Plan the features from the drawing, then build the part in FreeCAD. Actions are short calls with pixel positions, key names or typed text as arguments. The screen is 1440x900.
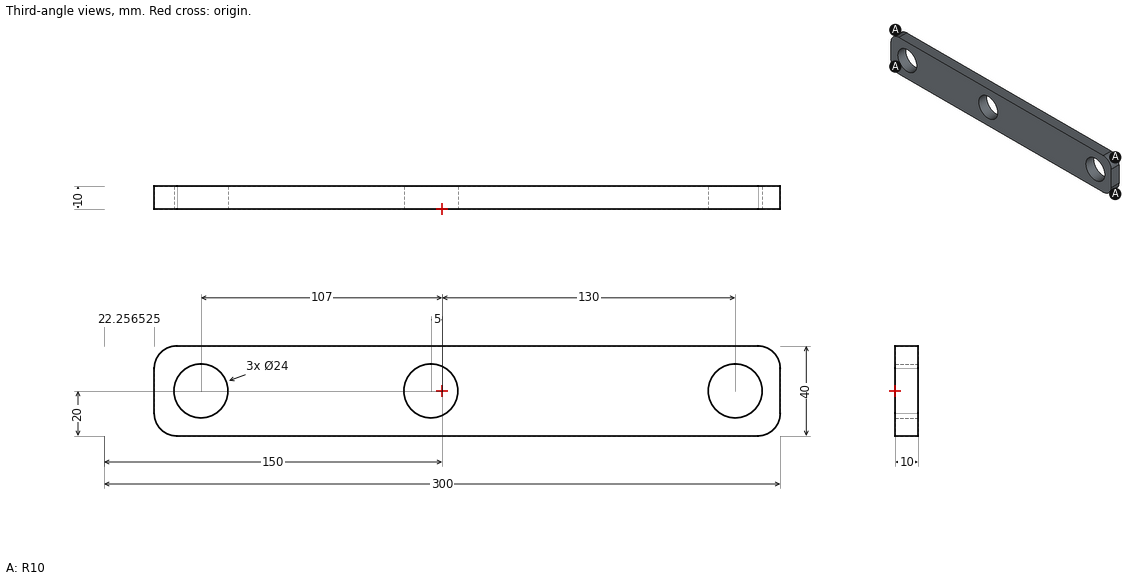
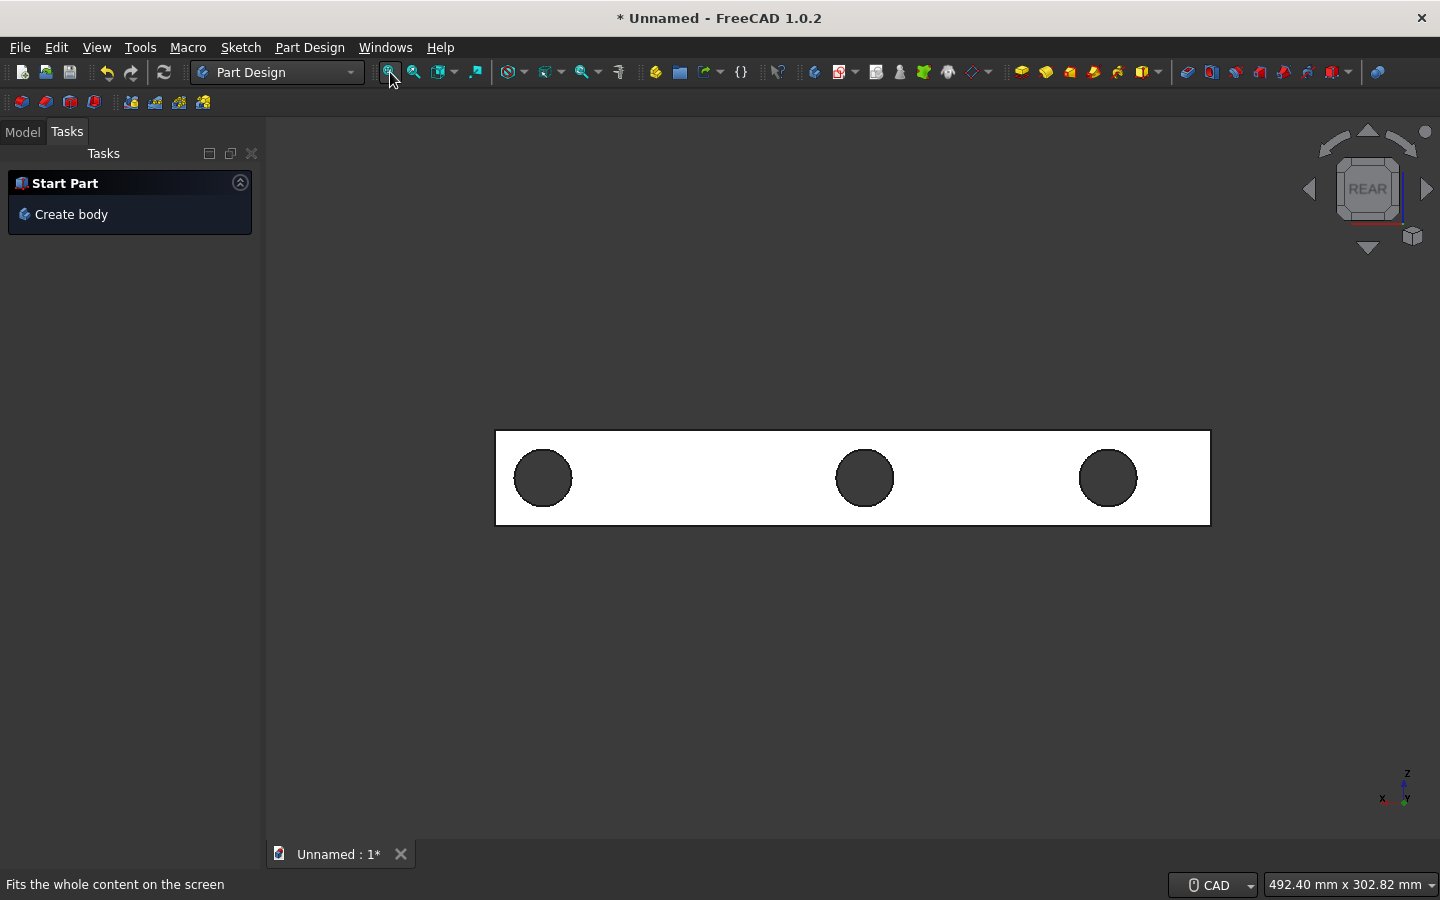
click(649, 477)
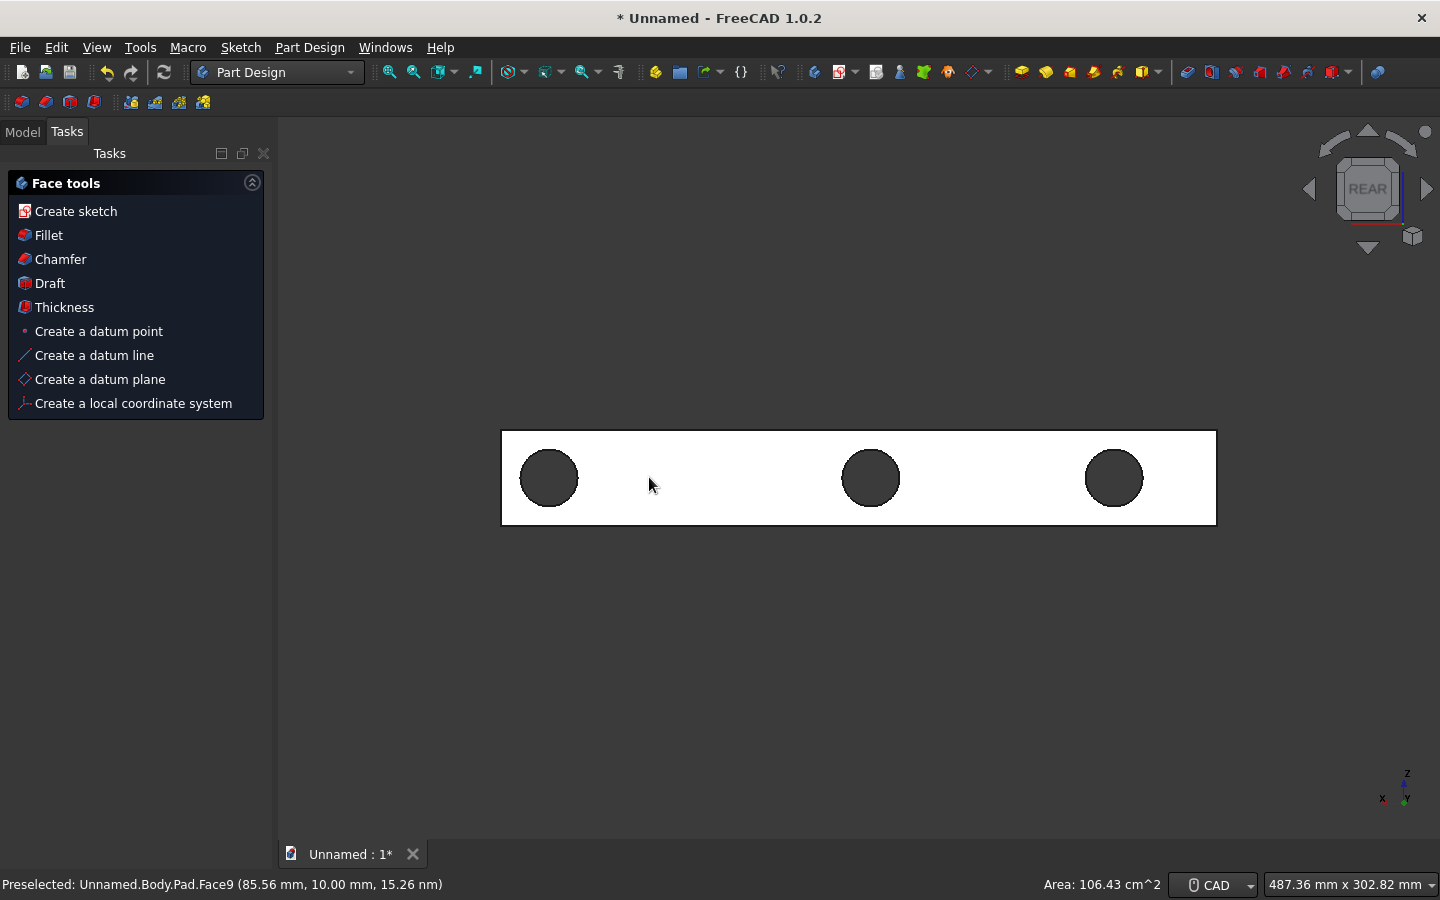
click(840, 72)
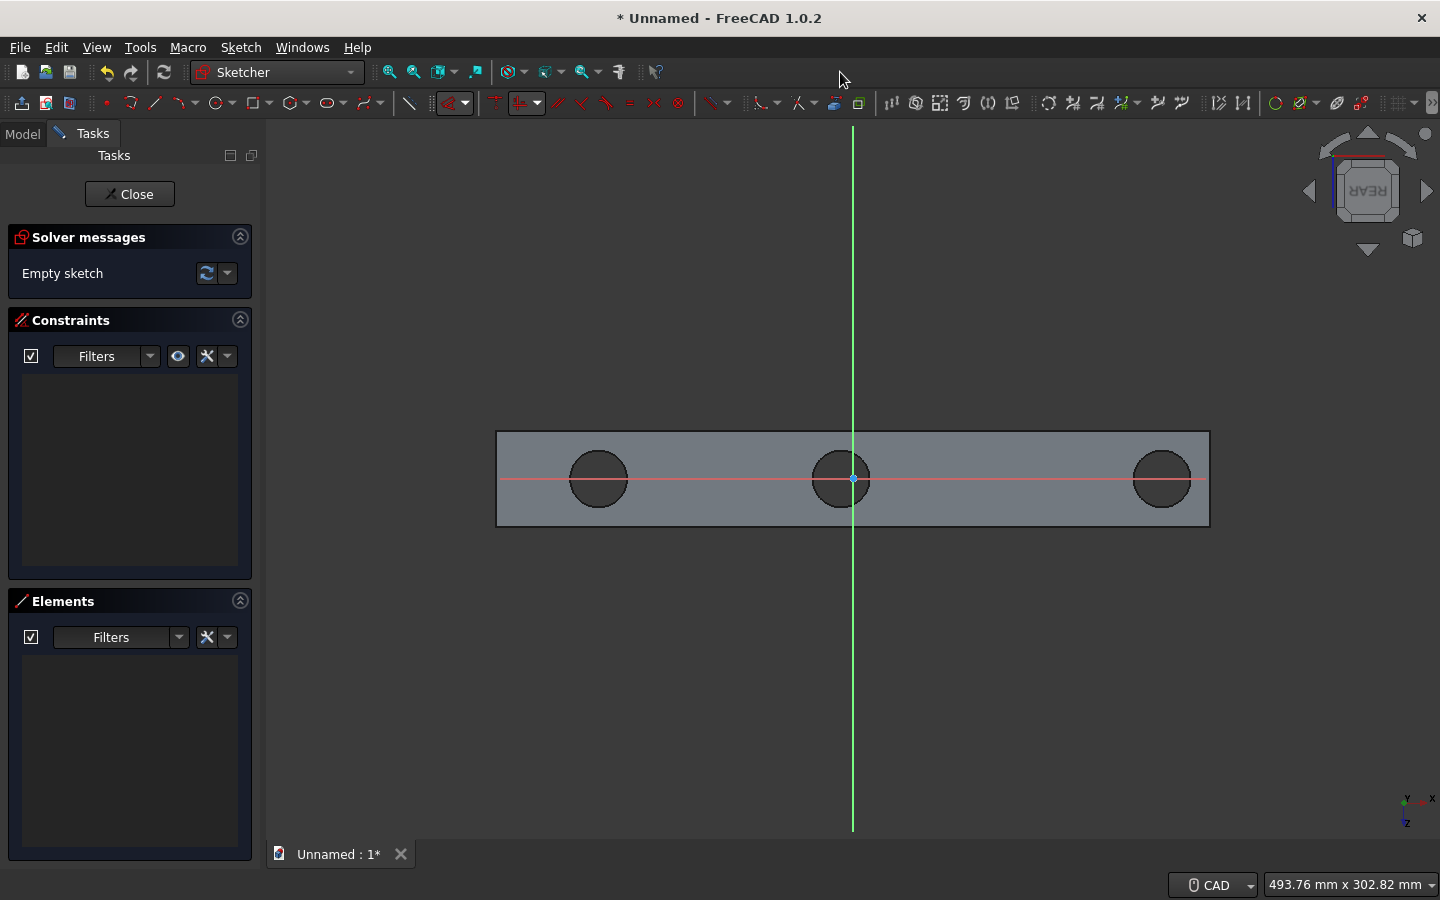
scroll(457, 479, up, 8)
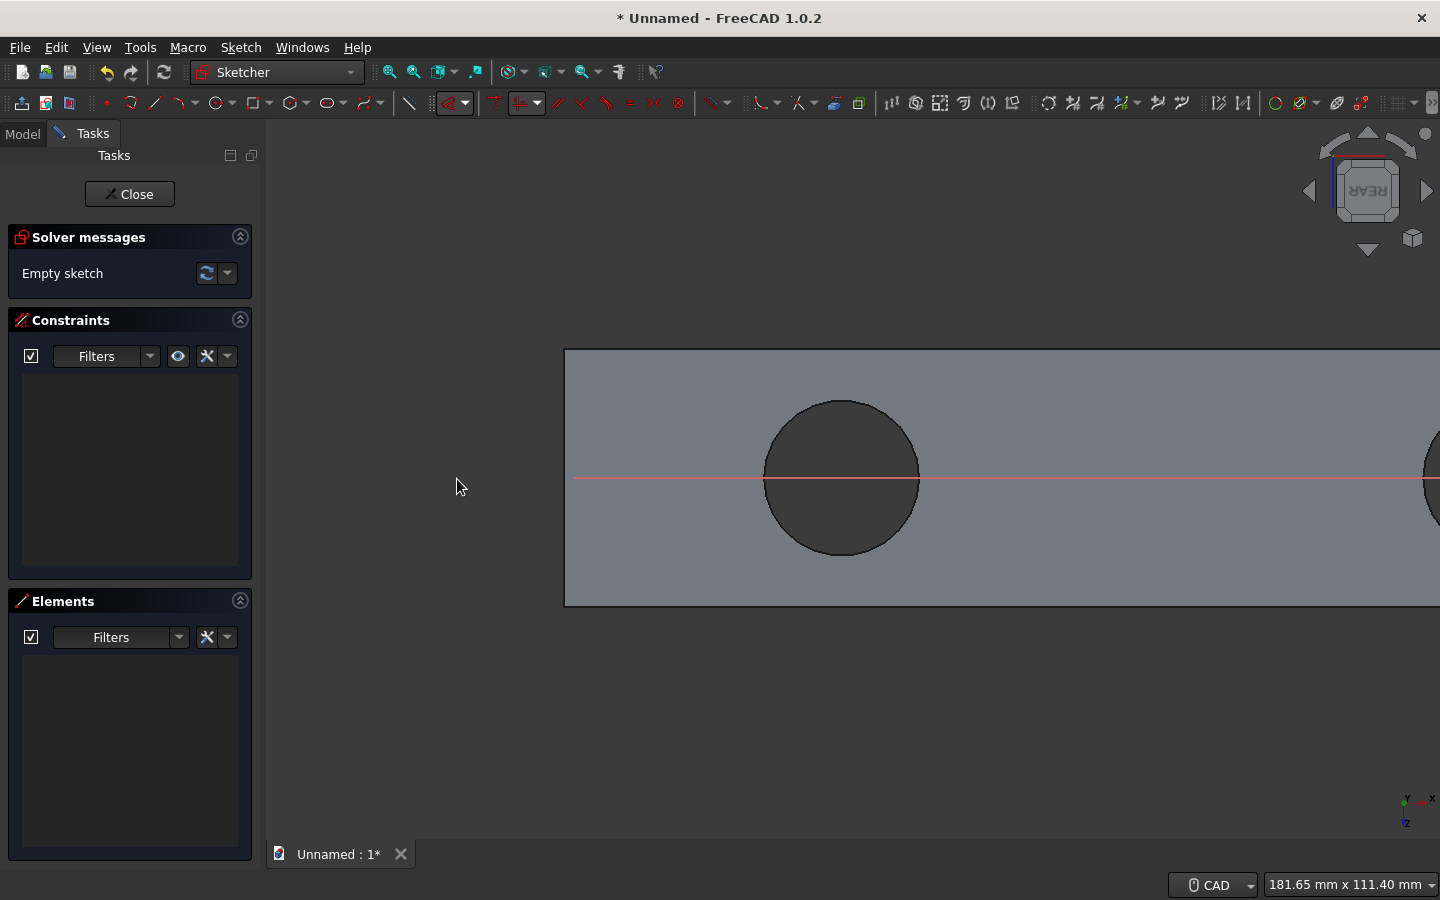
click(254, 104)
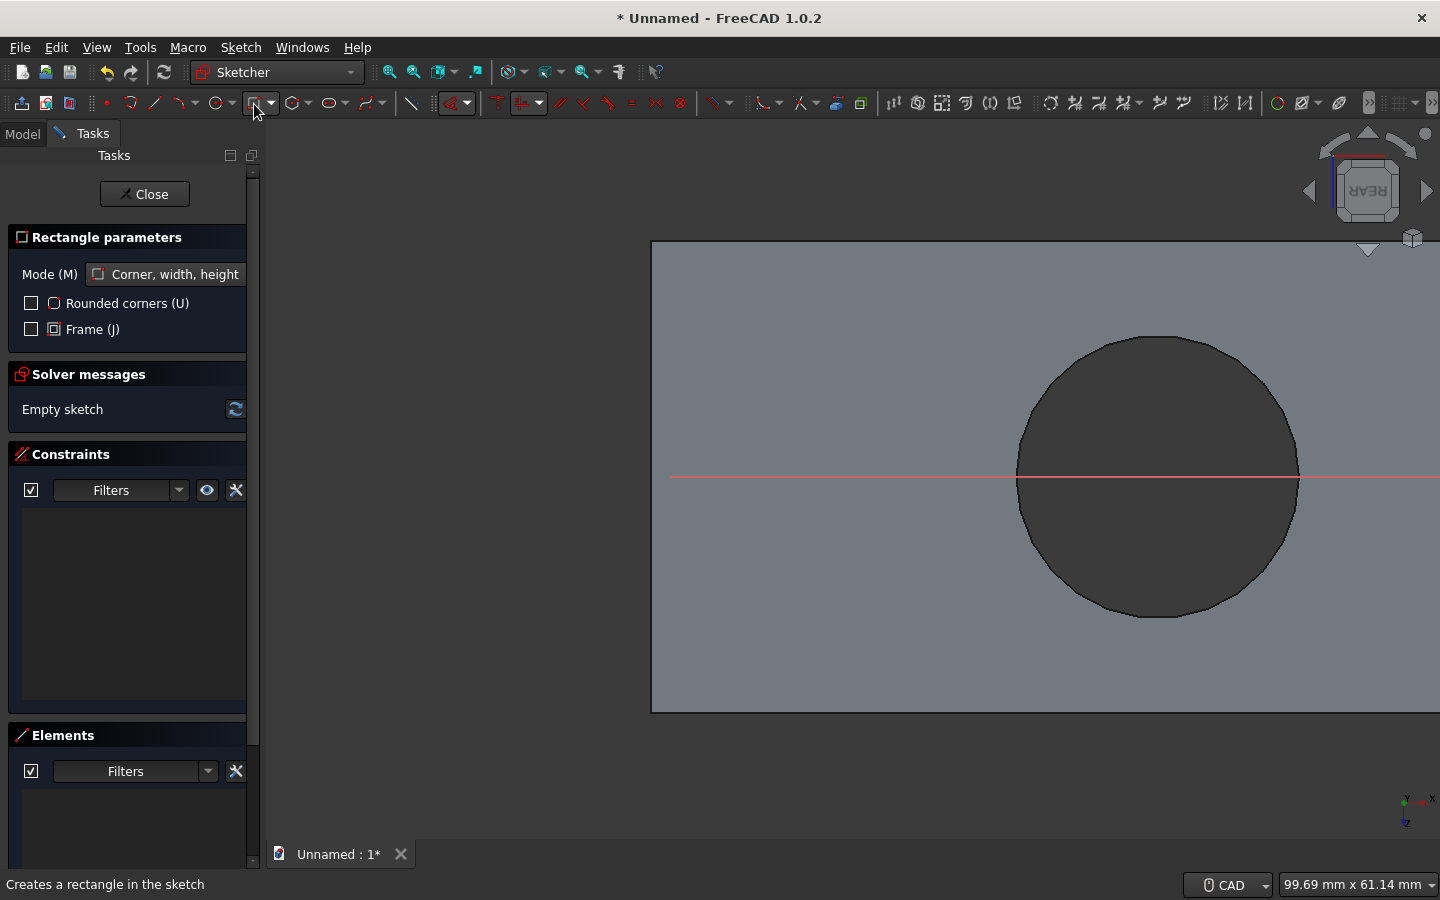
click(651, 241)
click(913, 713)
key(Escape)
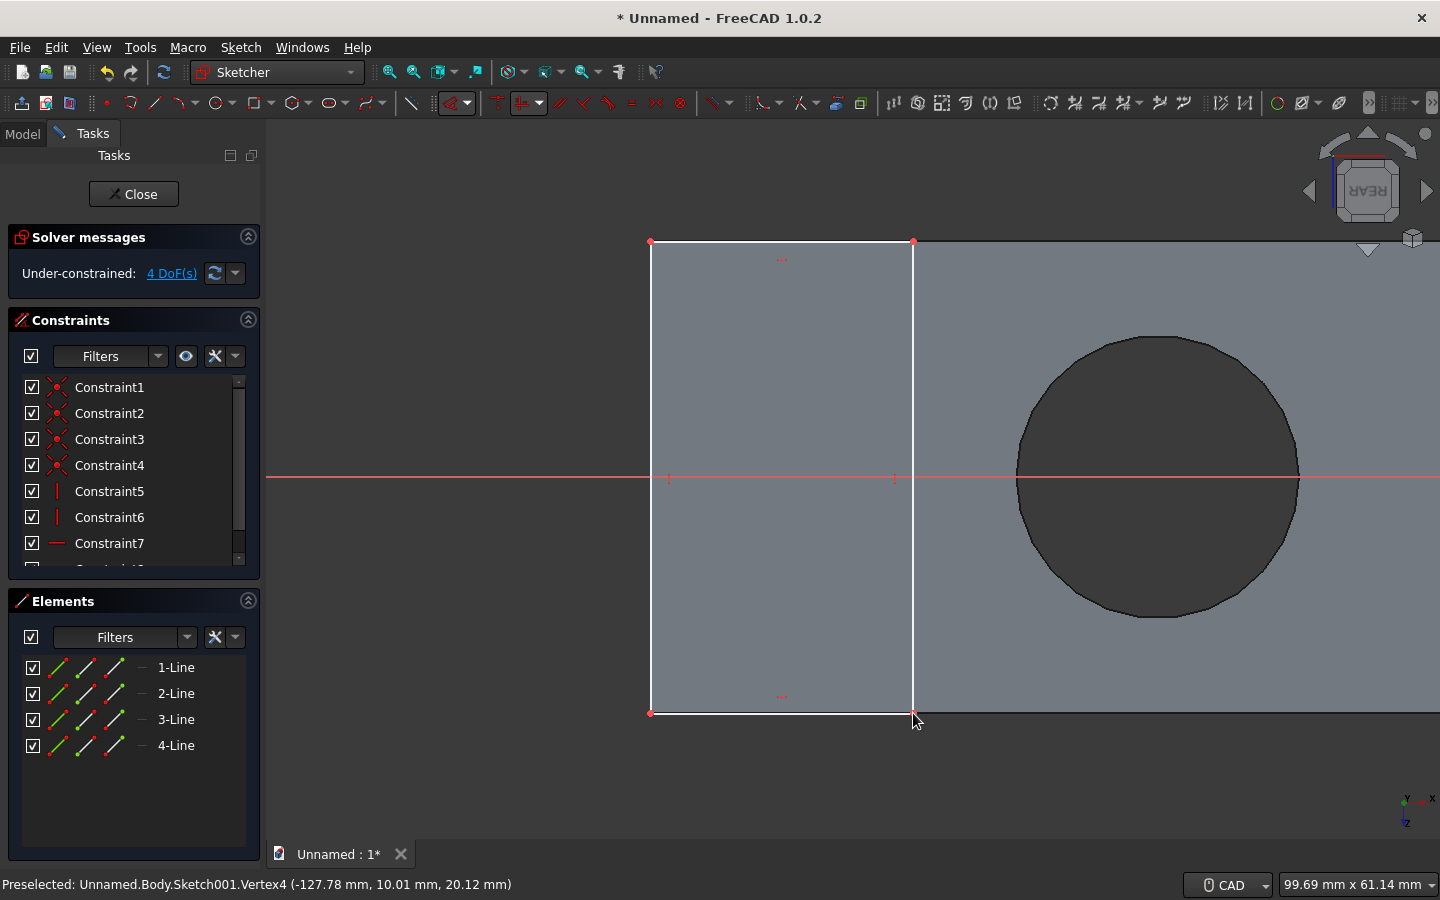
click(651, 384)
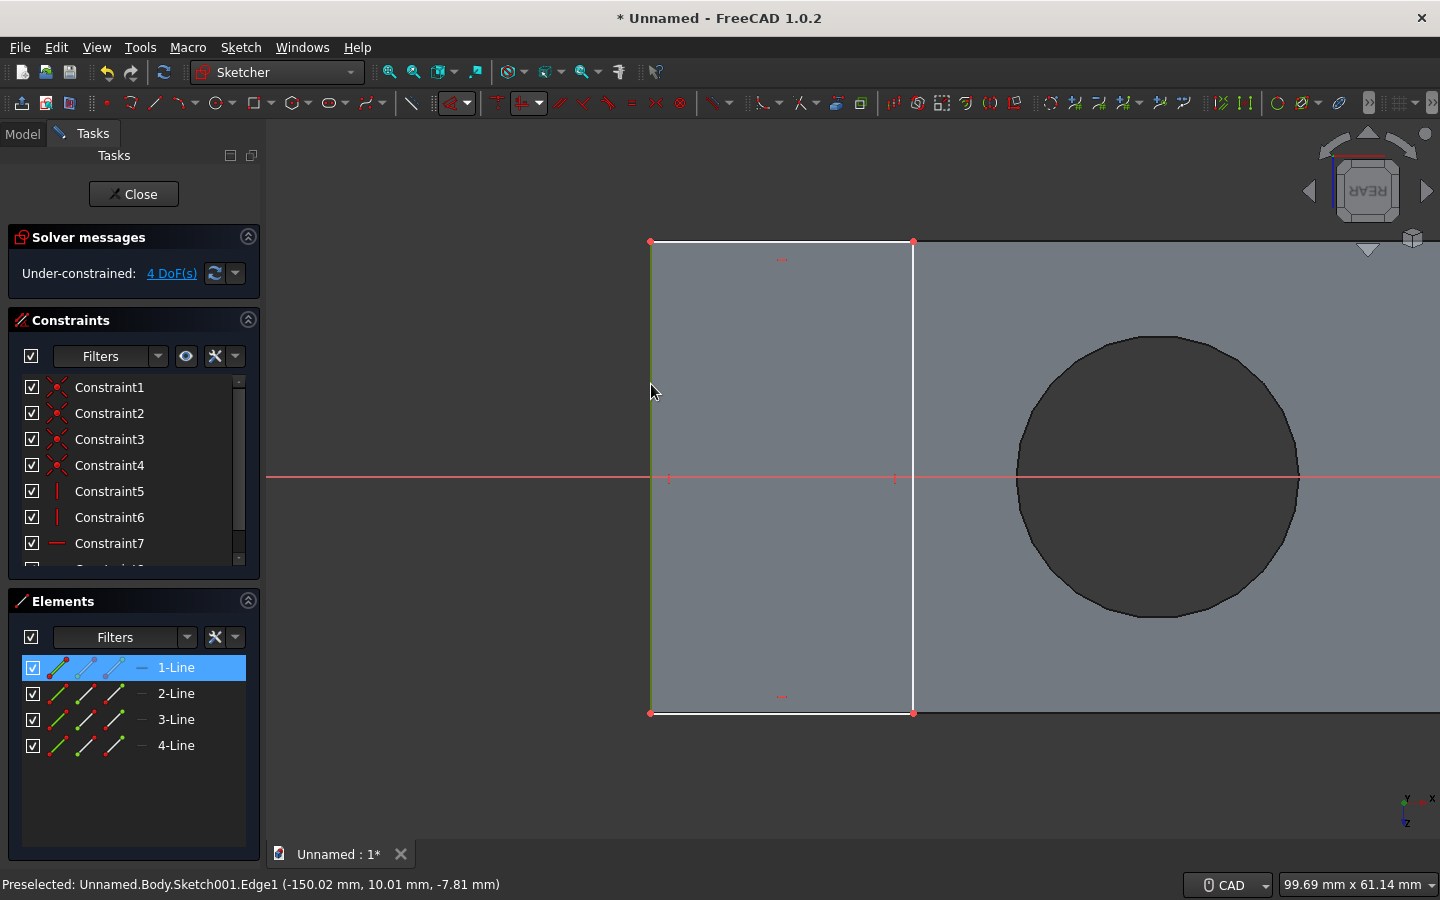
key(i)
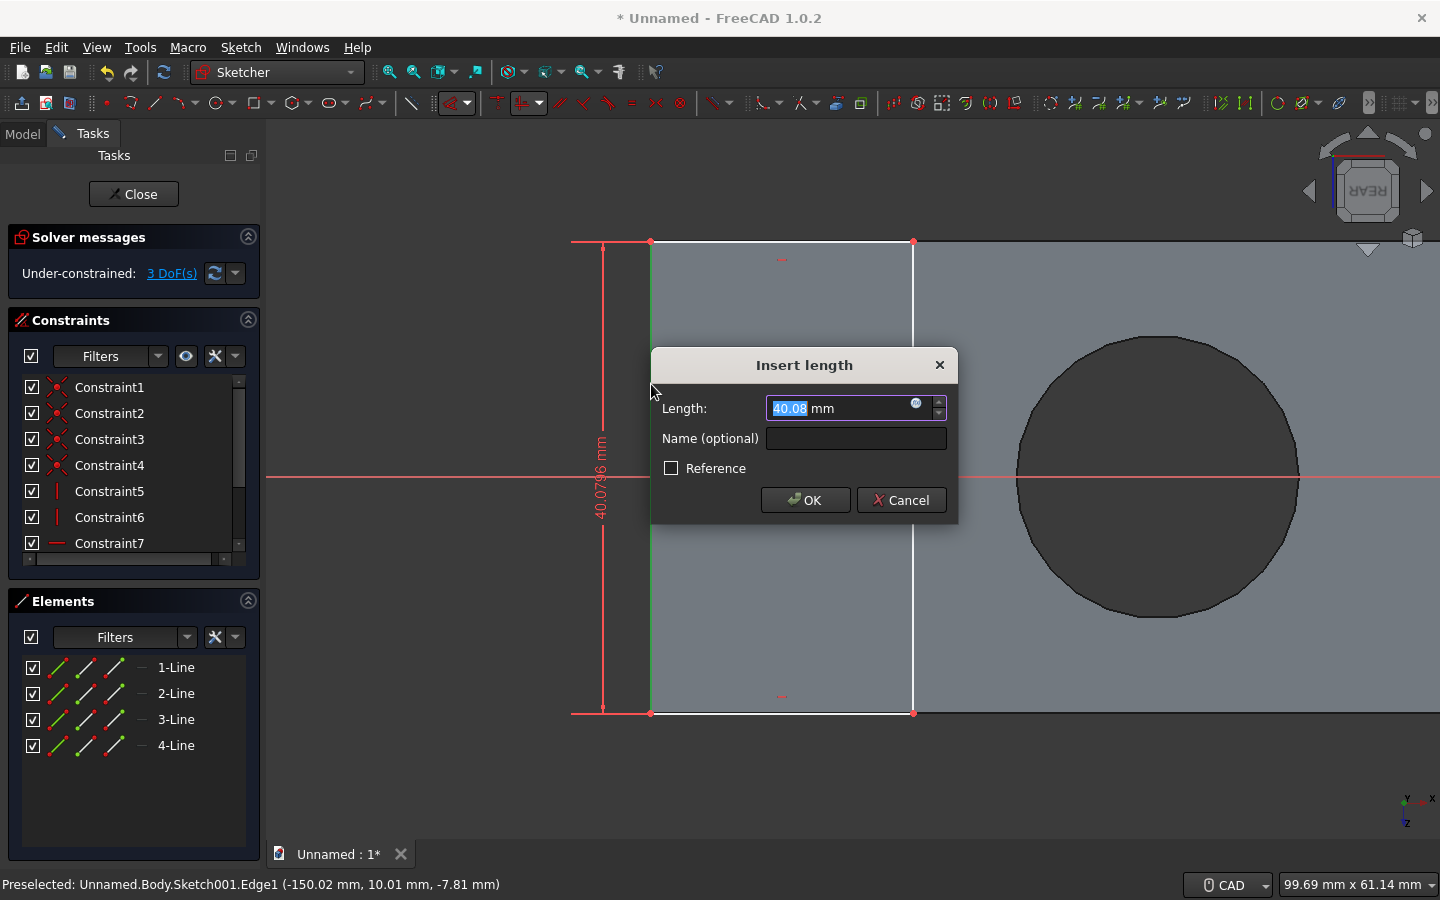
text(40)
key(Return)